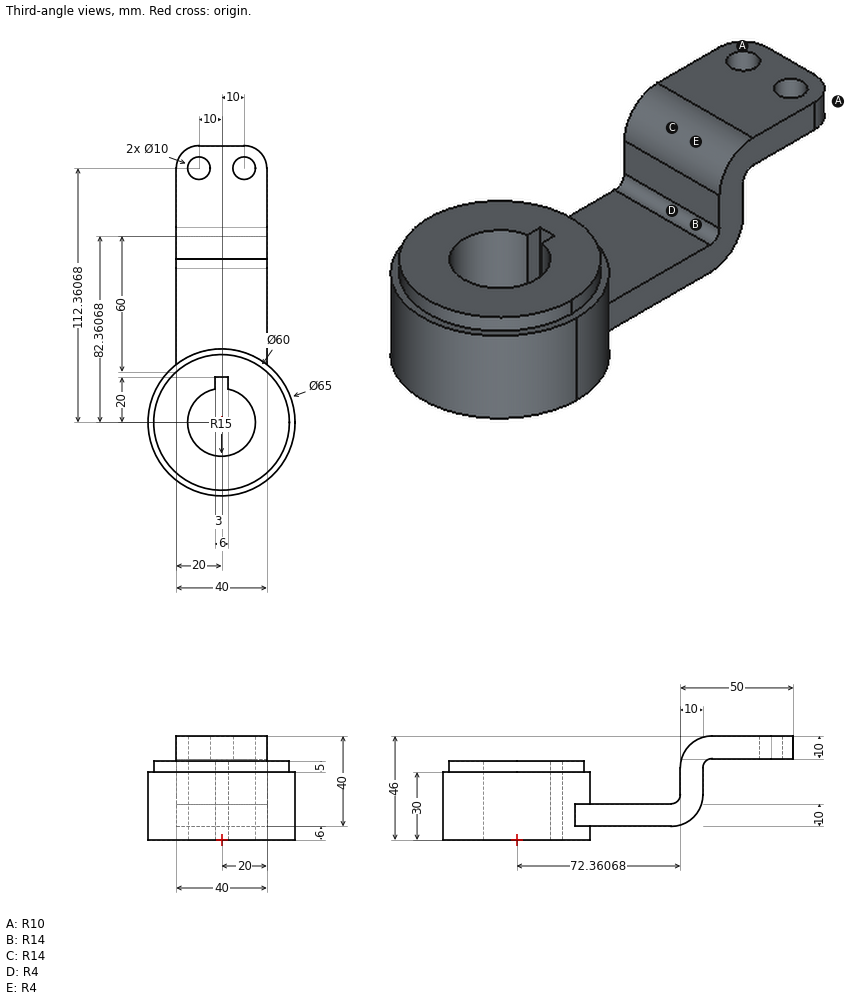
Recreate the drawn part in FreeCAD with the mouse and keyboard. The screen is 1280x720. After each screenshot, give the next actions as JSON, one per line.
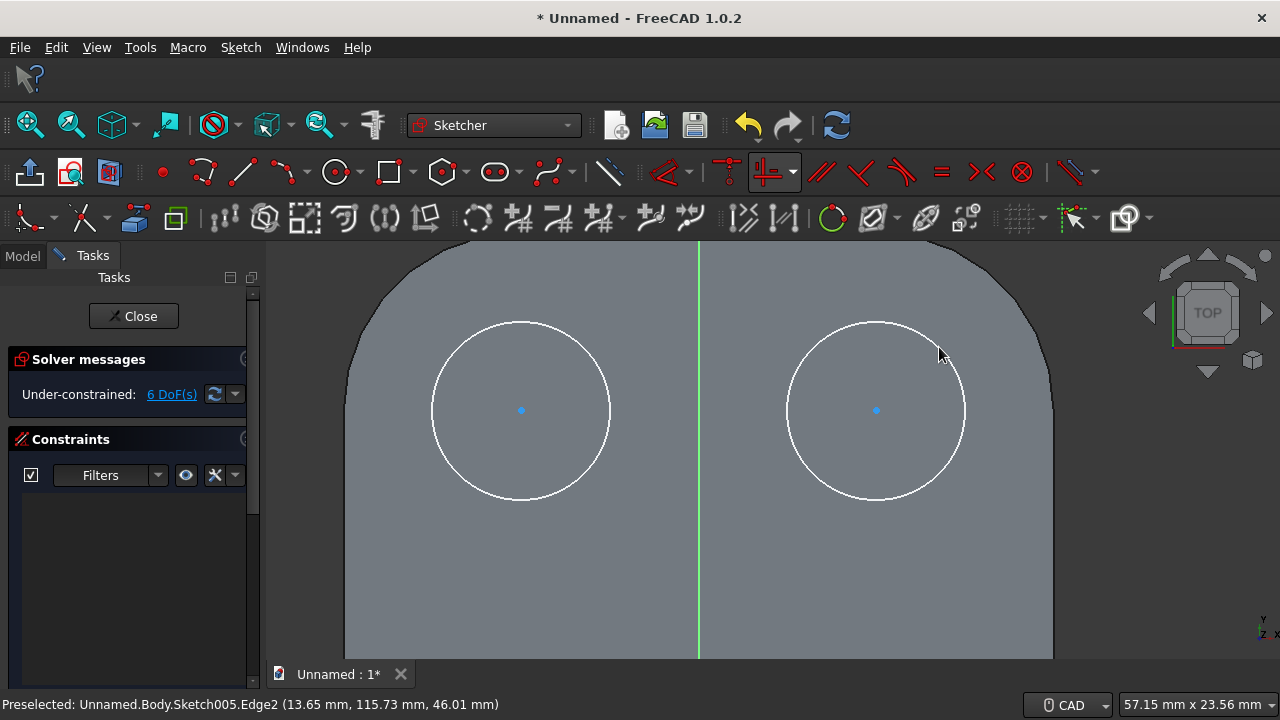
{"action": "left_click", "coordinate": [584, 348]}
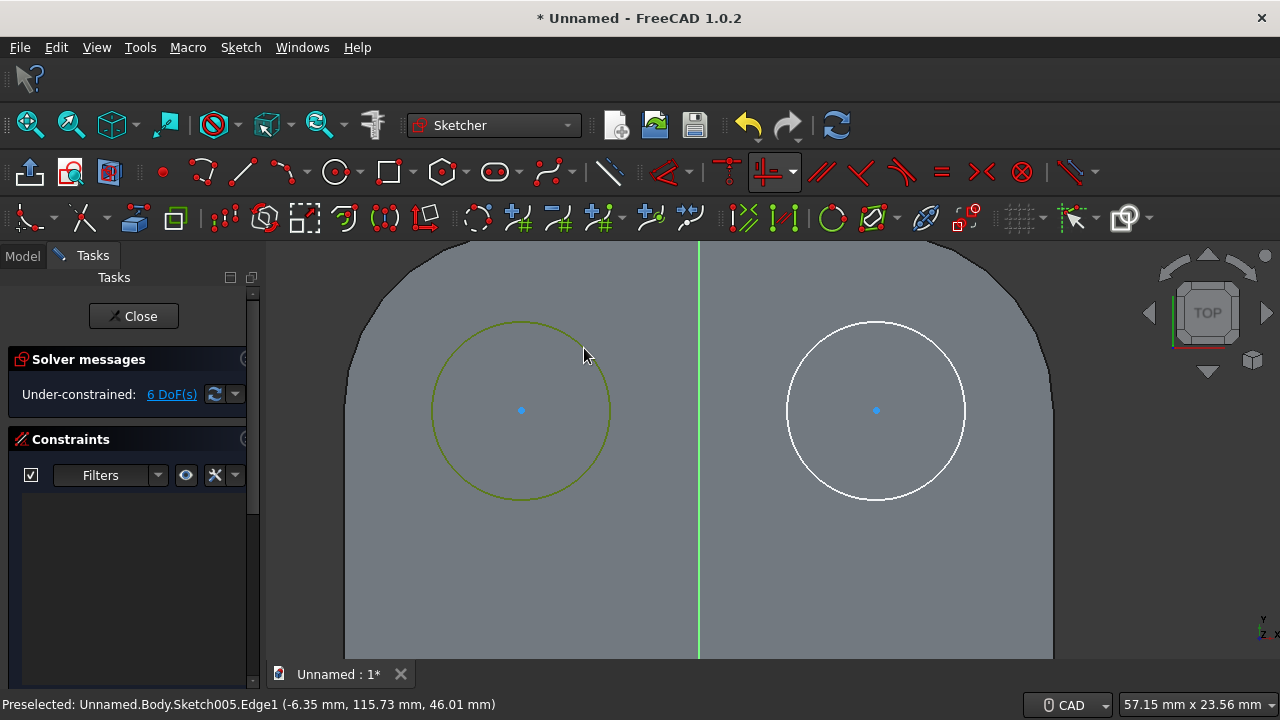
{"action": "left_click", "coordinate": [939, 348]}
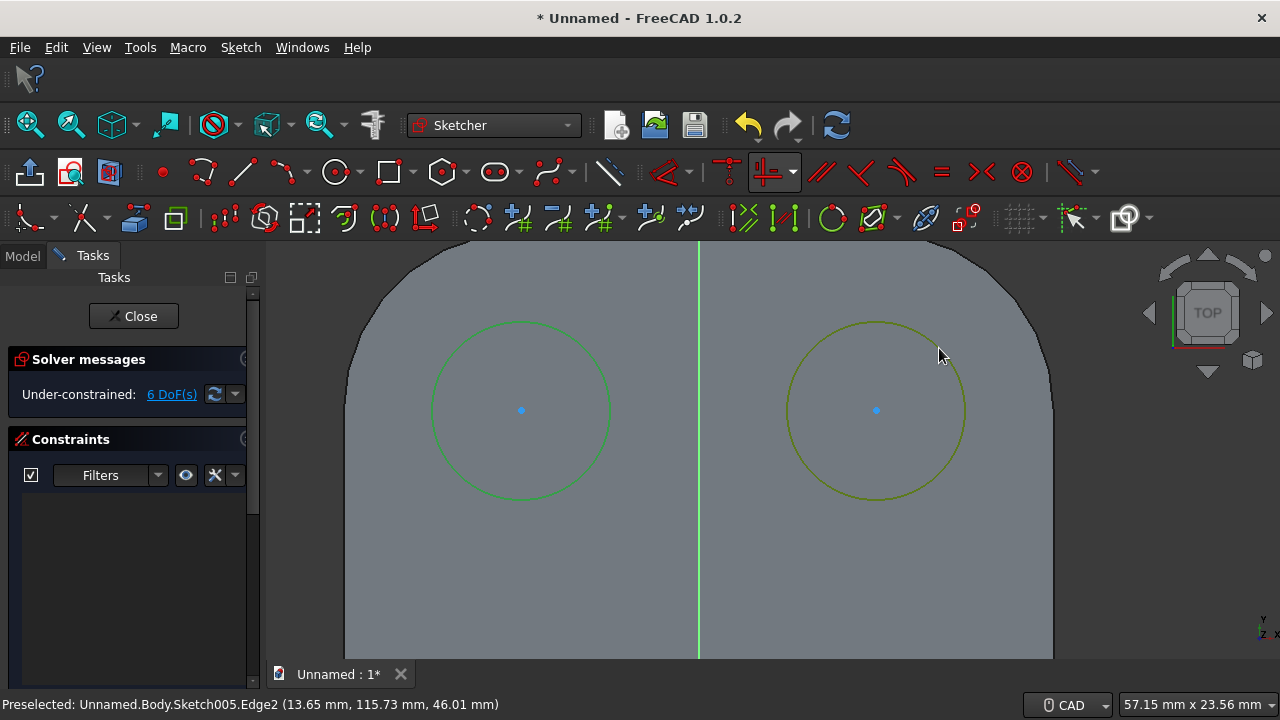
{"action": "key", "text": "e"}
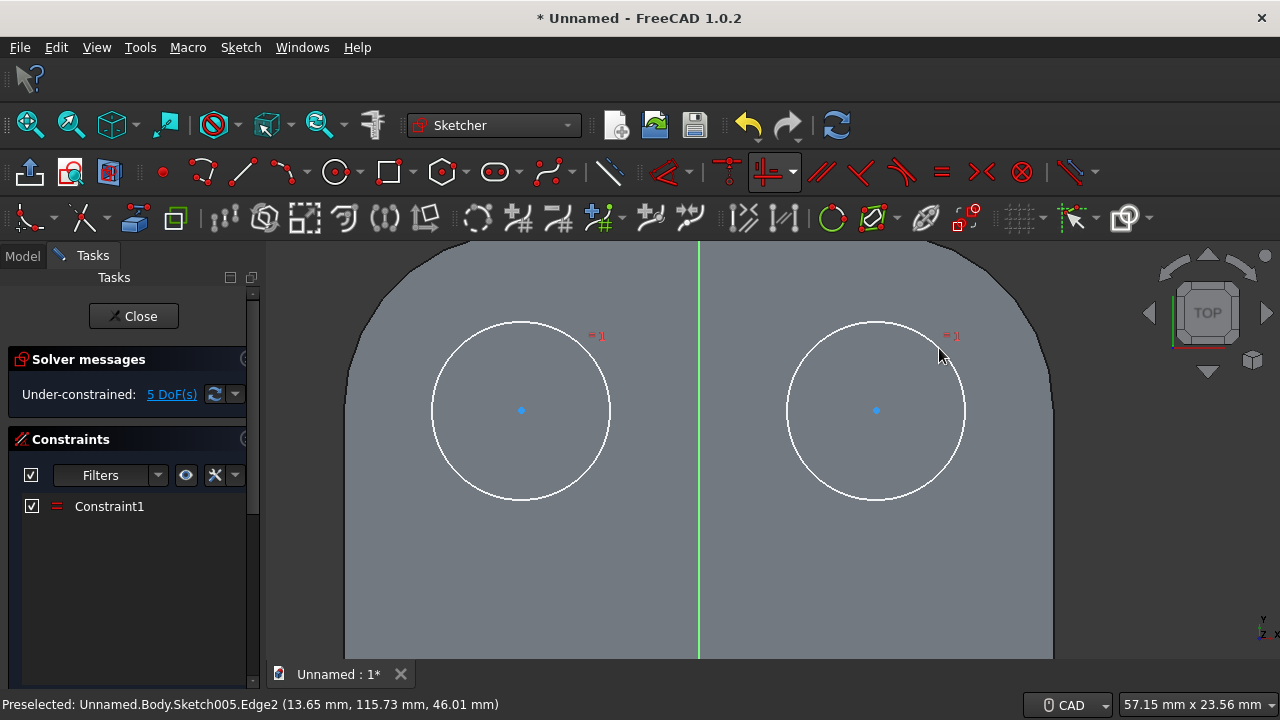
{"action": "left_click", "coordinate": [521, 411]}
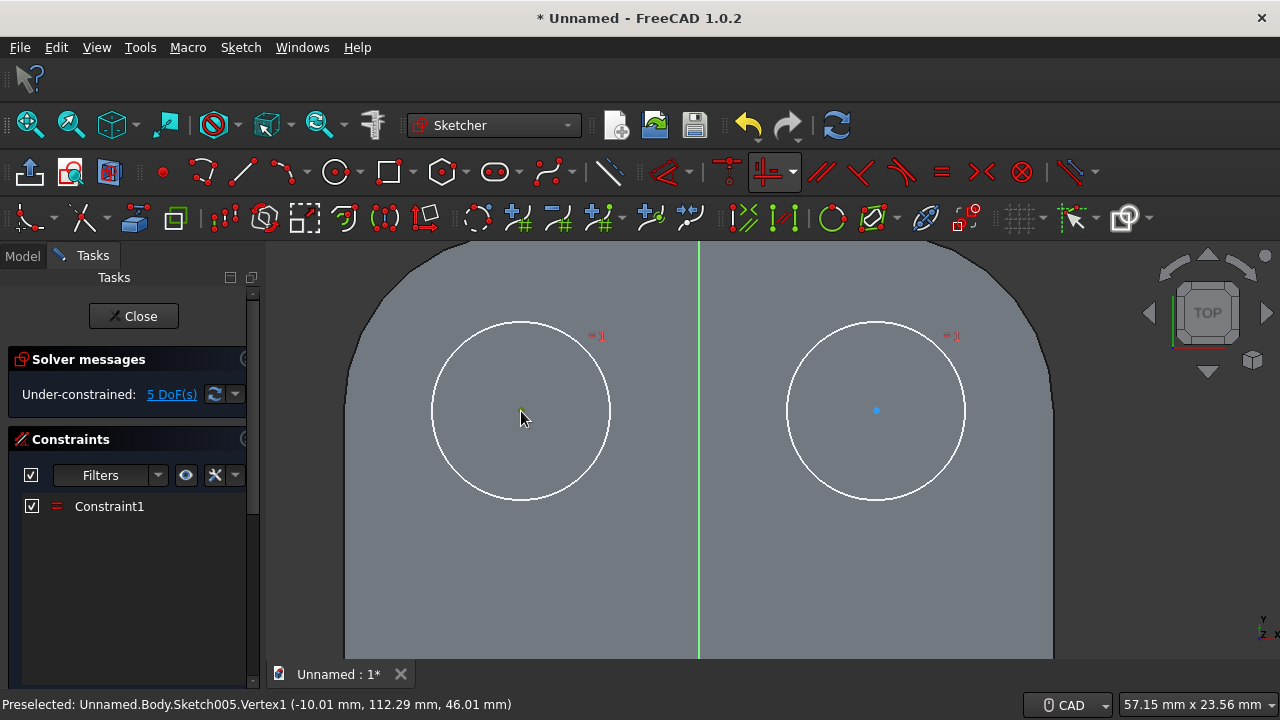
{"action": "left_click", "coordinate": [876, 411]}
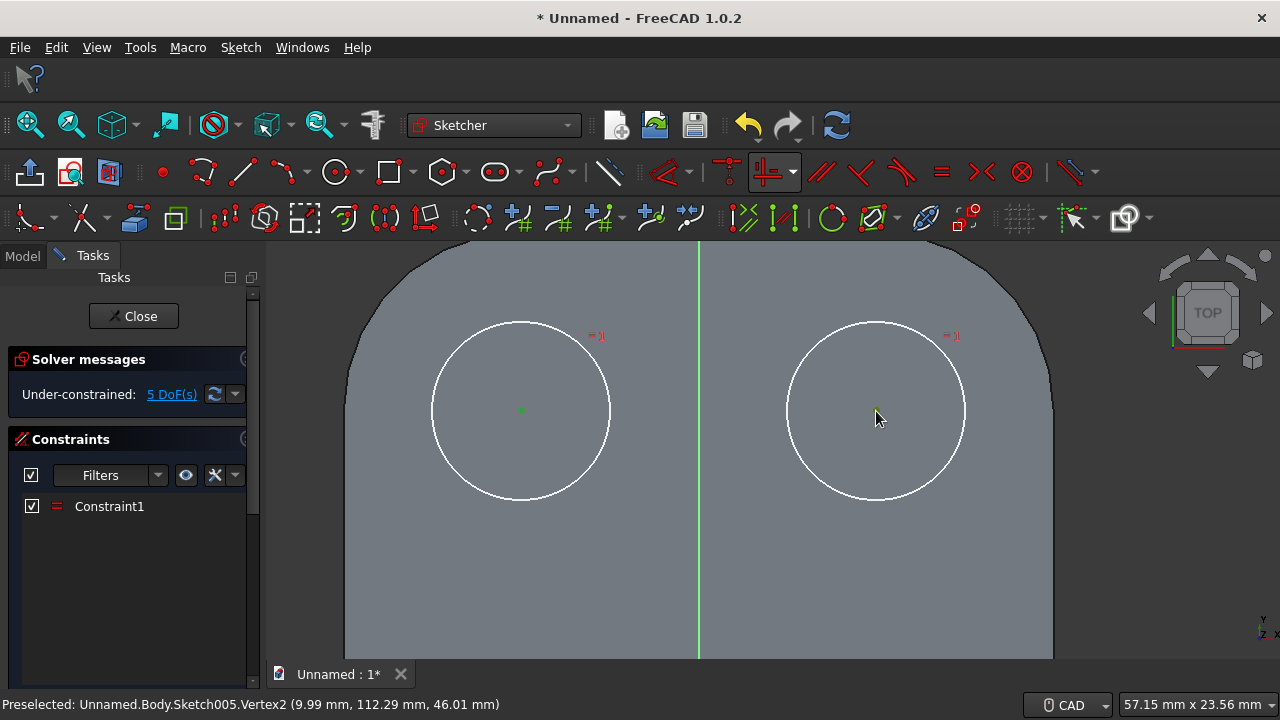
{"action": "left_click", "coordinate": [796, 172]}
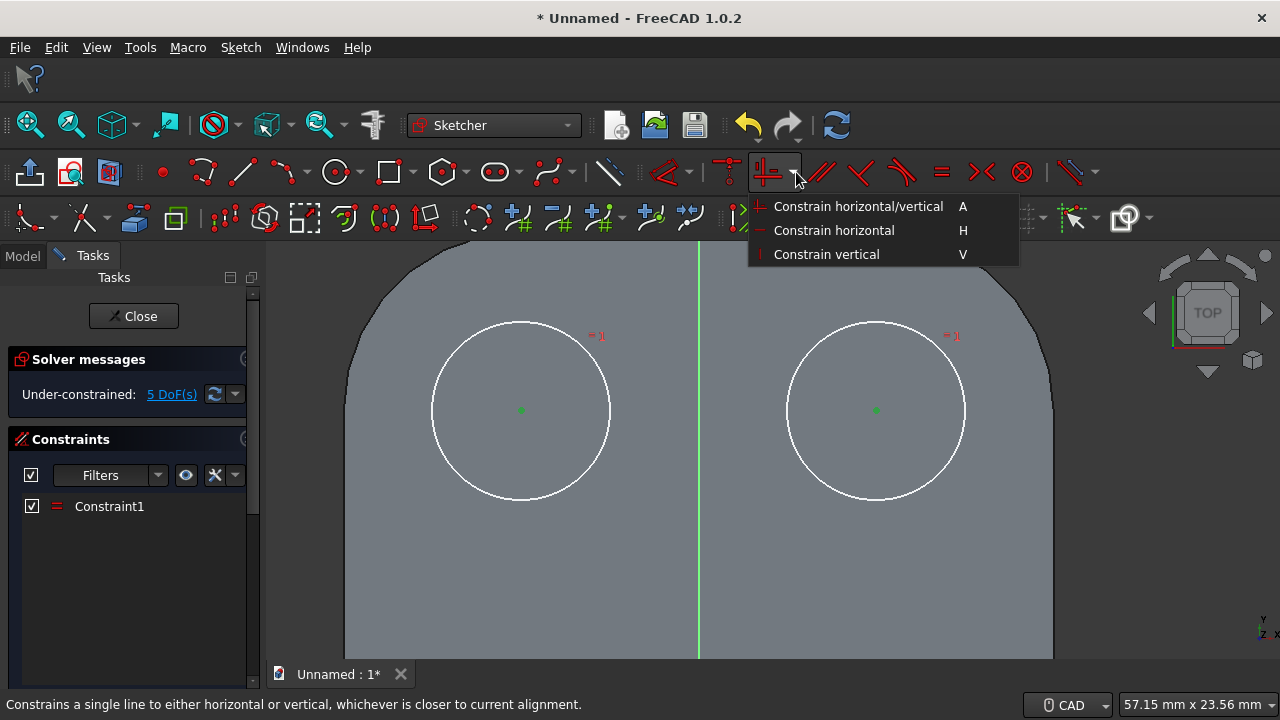
{"action": "left_click", "coordinate": [884, 230]}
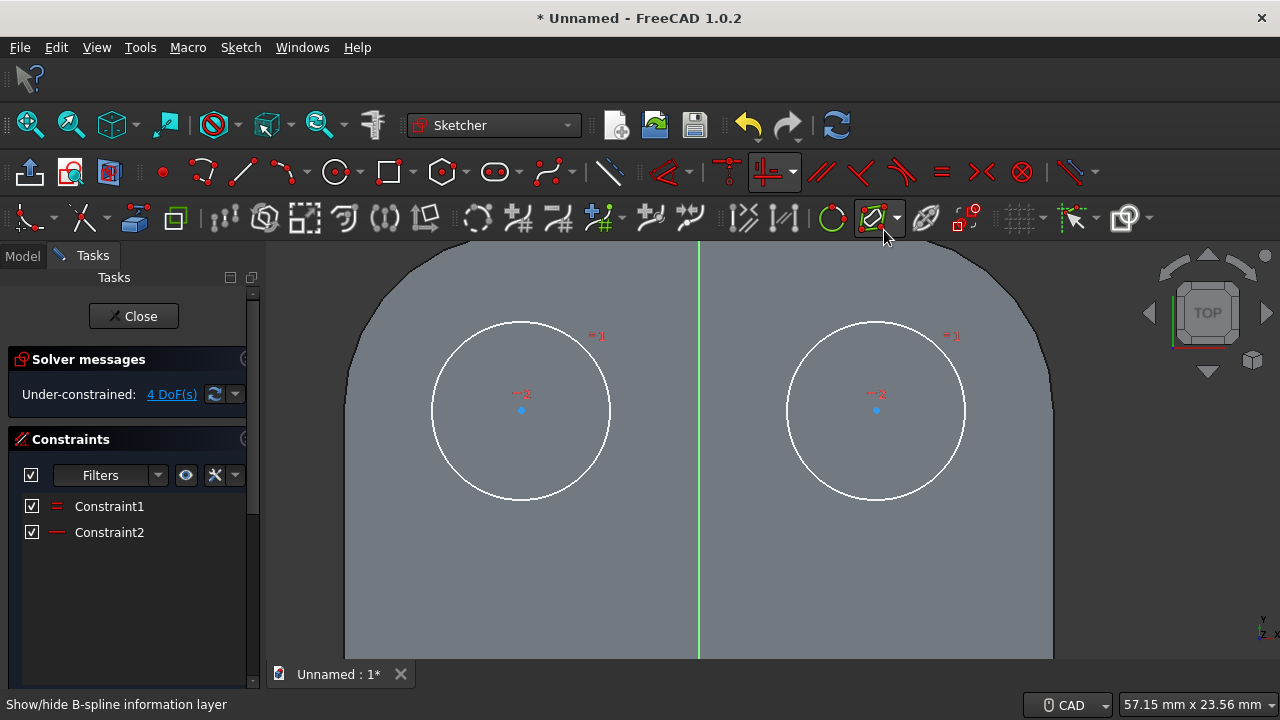
{"action": "key", "text": "d"}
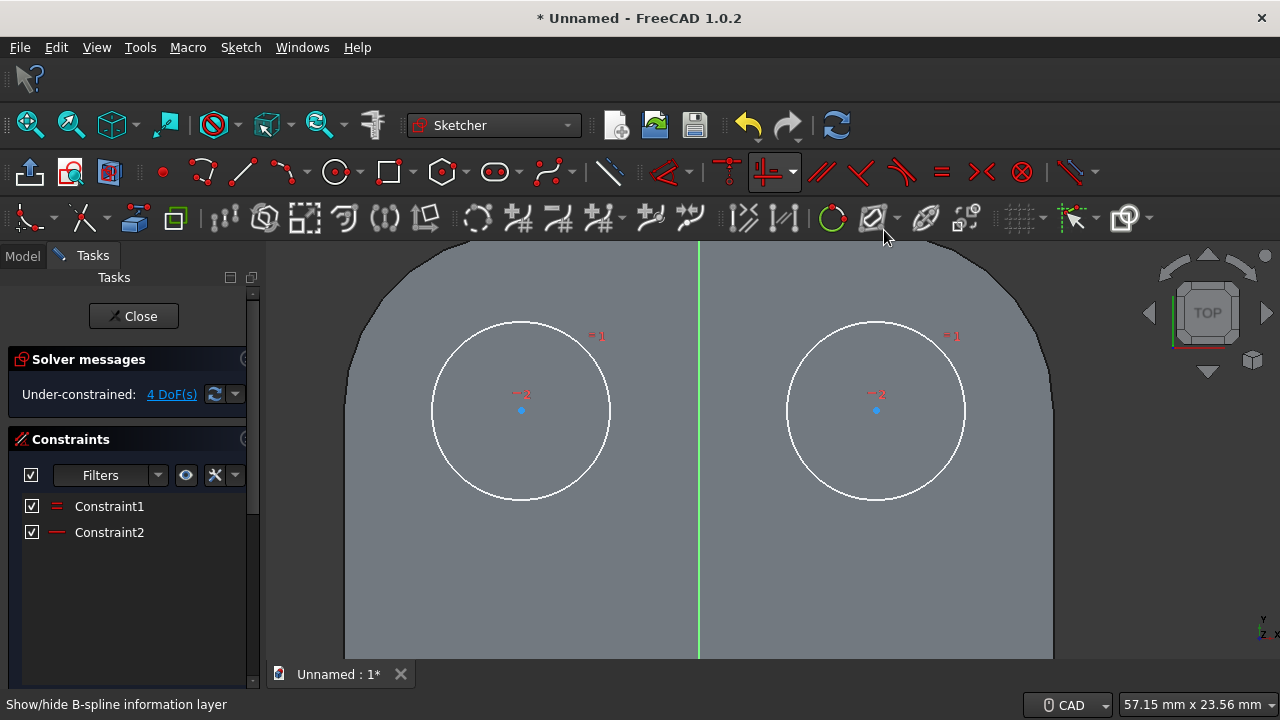
{"action": "left_click", "coordinate": [584, 348]}
{"action": "left_click", "coordinate": [607, 325]}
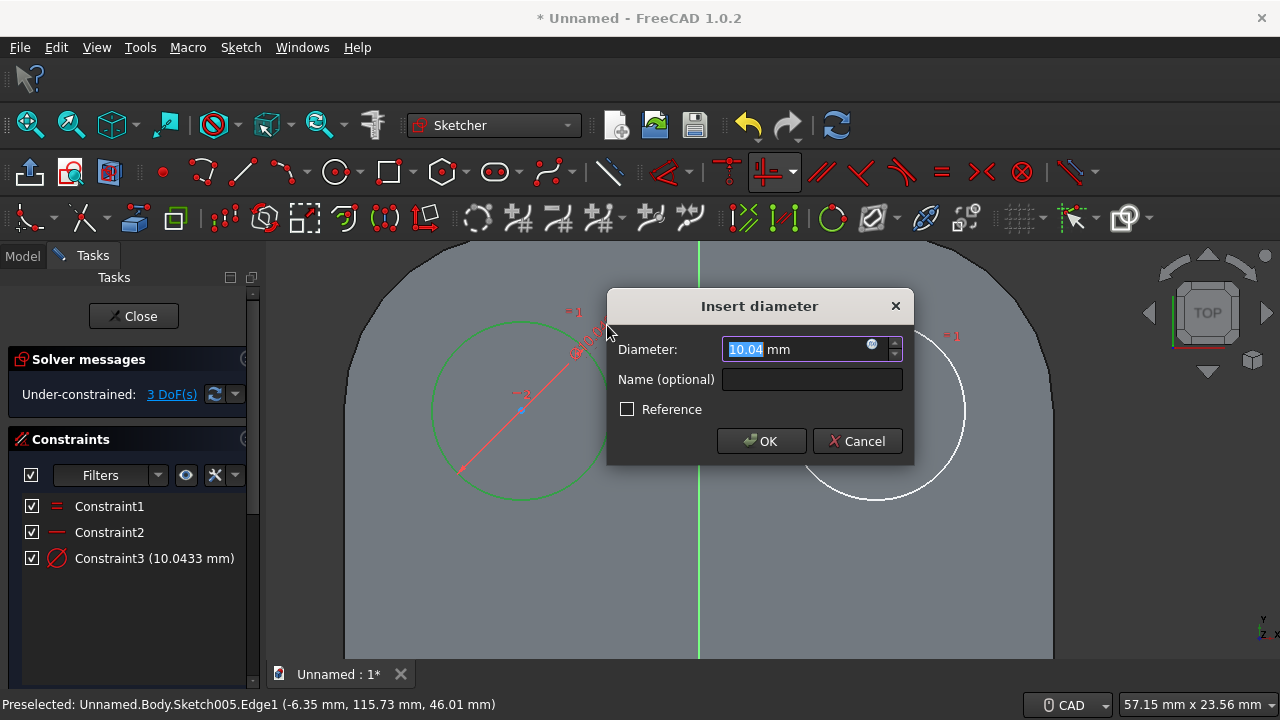
{"action": "type", "text": "10"}
{"action": "key", "text": "Return"}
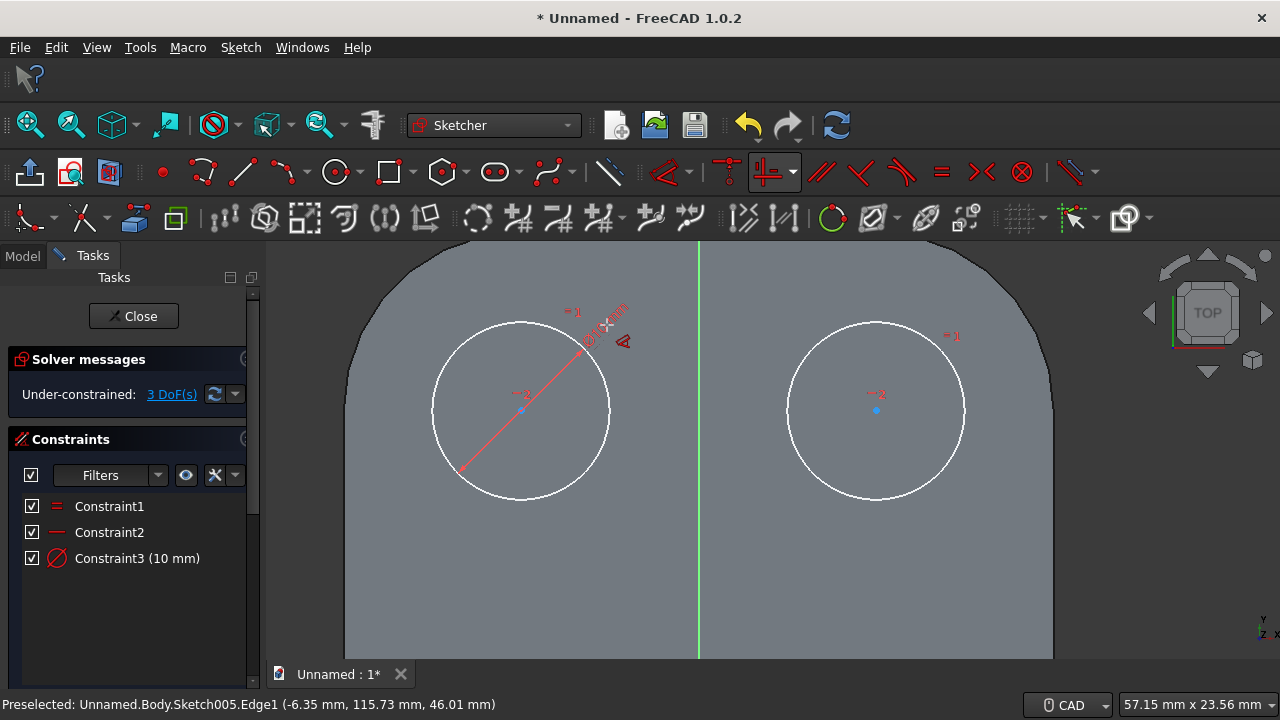
{"action": "left_click", "coordinate": [521, 411]}
{"action": "left_click", "coordinate": [569, 377]}